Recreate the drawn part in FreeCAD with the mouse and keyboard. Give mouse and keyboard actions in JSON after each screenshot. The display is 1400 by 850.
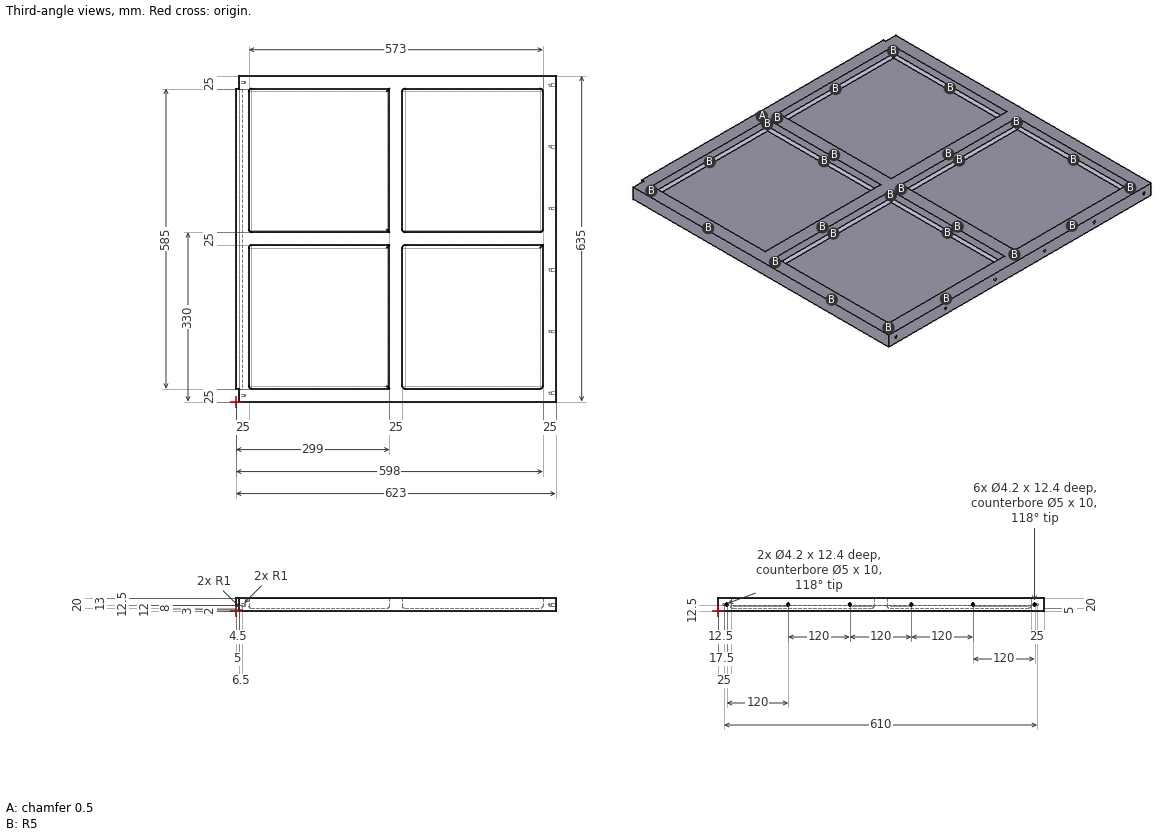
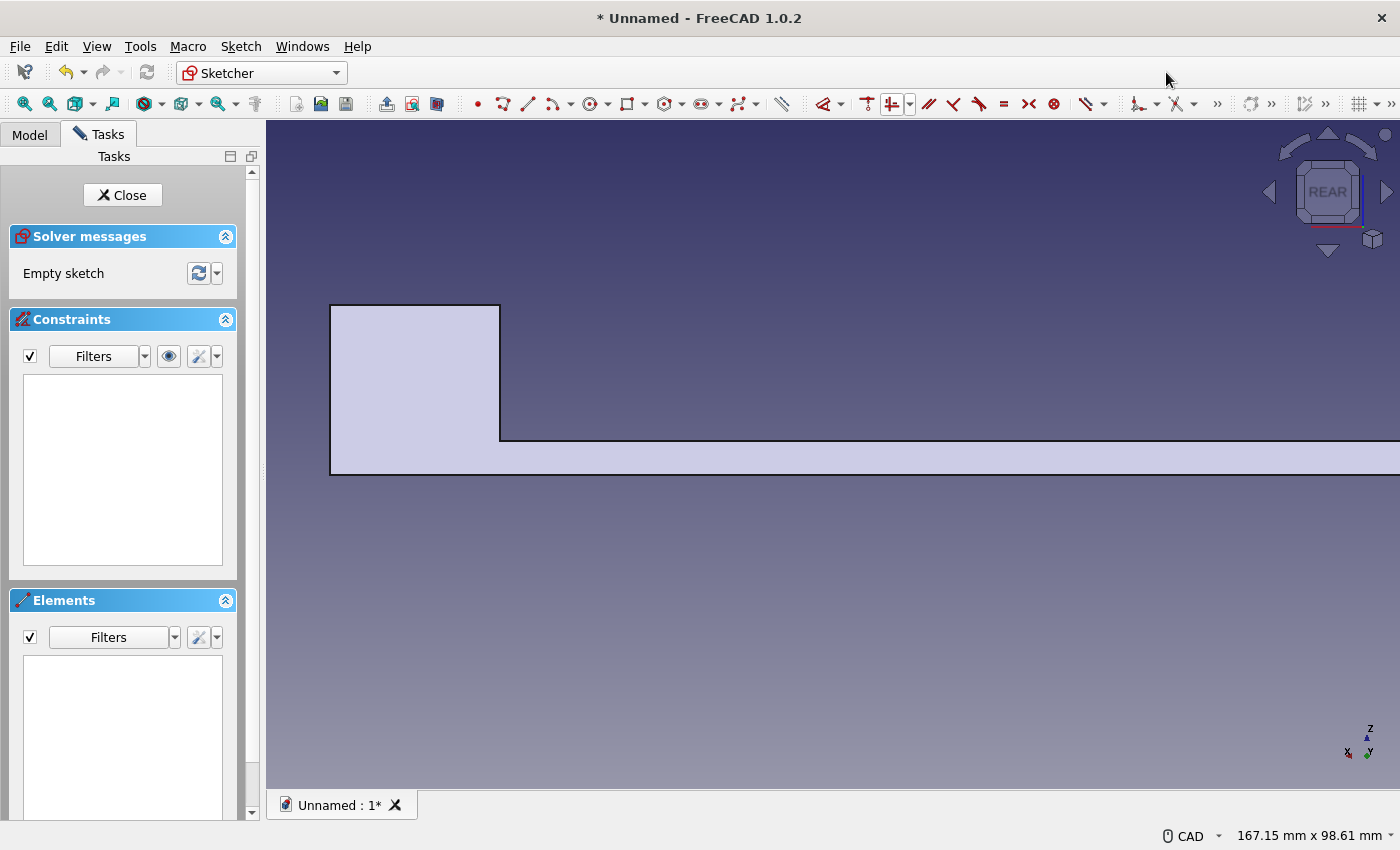
{"action": "scroll", "coordinate": [764, 454], "scroll_direction": "down", "scroll_amount": 5}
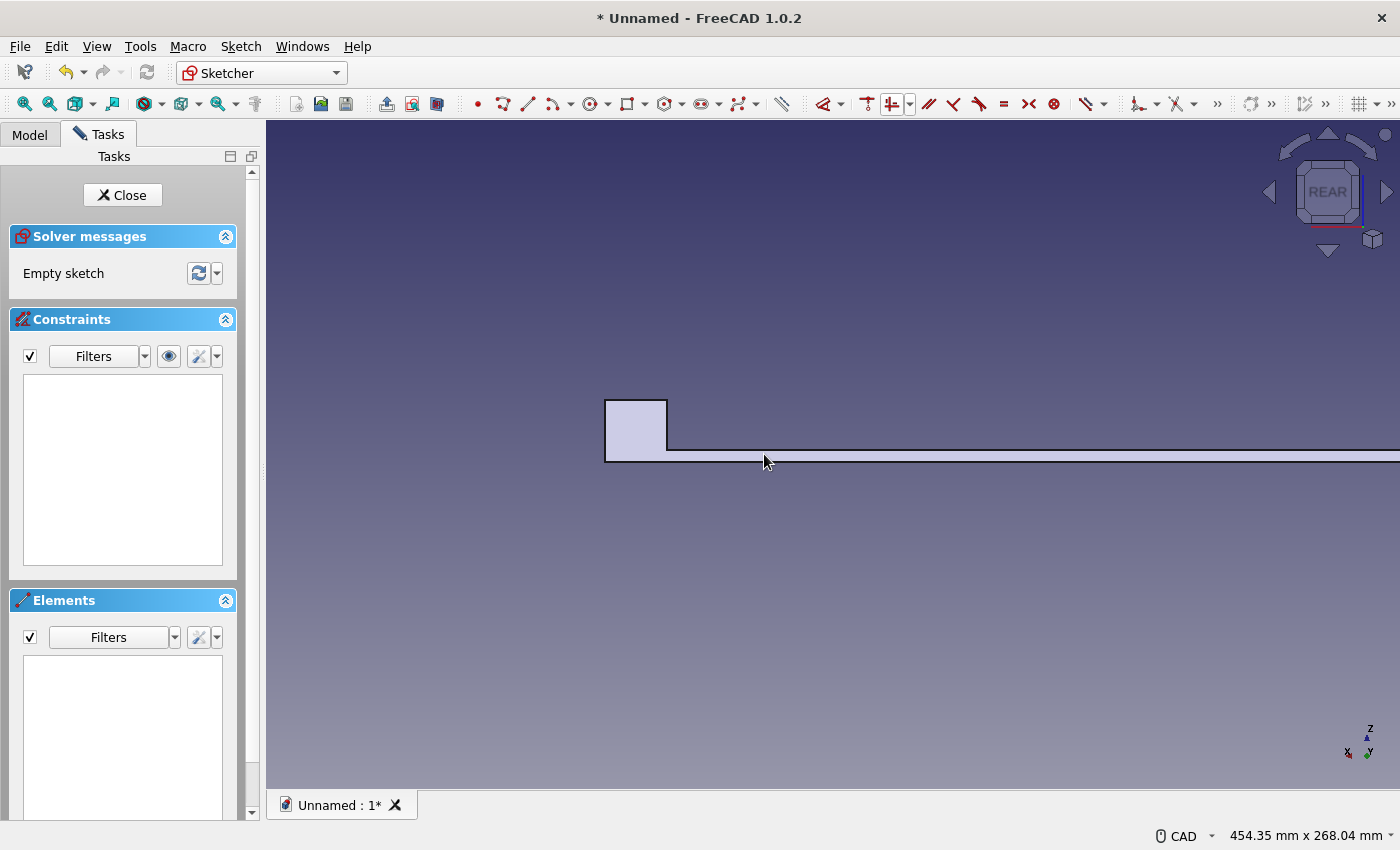
{"action": "scroll", "coordinate": [764, 454], "scroll_direction": "down", "scroll_amount": 5}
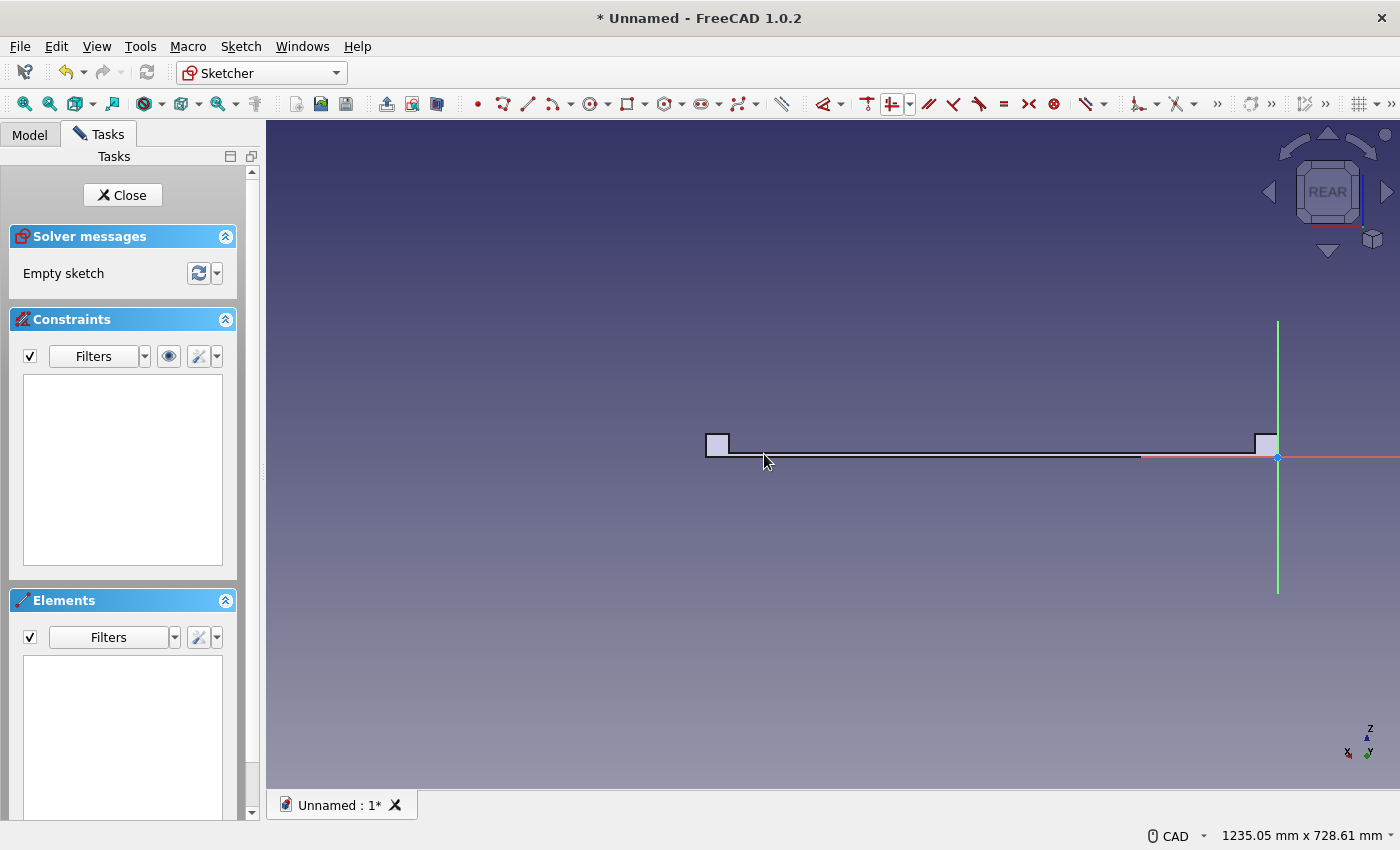
{"action": "scroll", "coordinate": [764, 454], "scroll_direction": "down", "scroll_amount": 5}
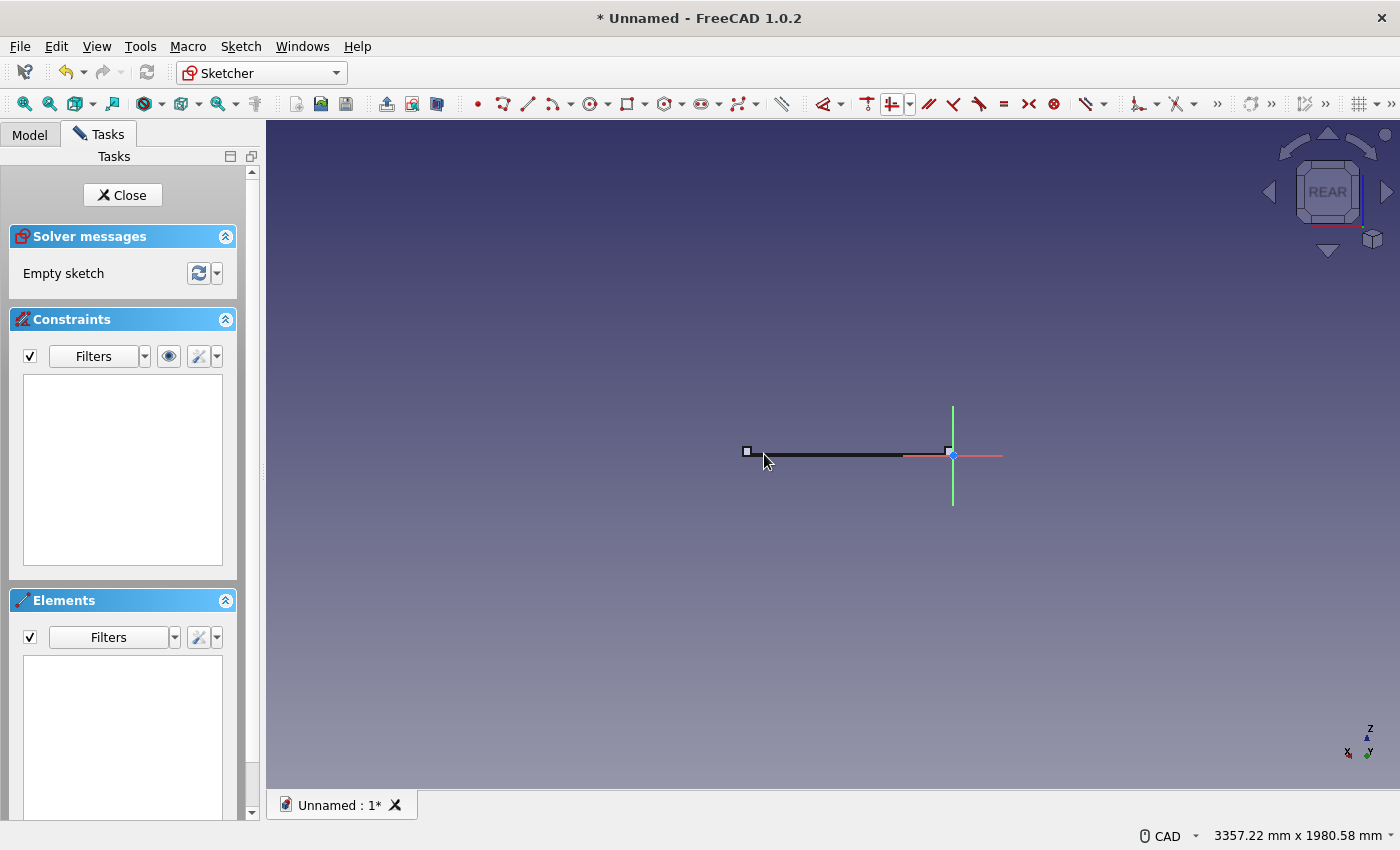
{"action": "scroll", "coordinate": [961, 453], "scroll_direction": "up", "scroll_amount": 15}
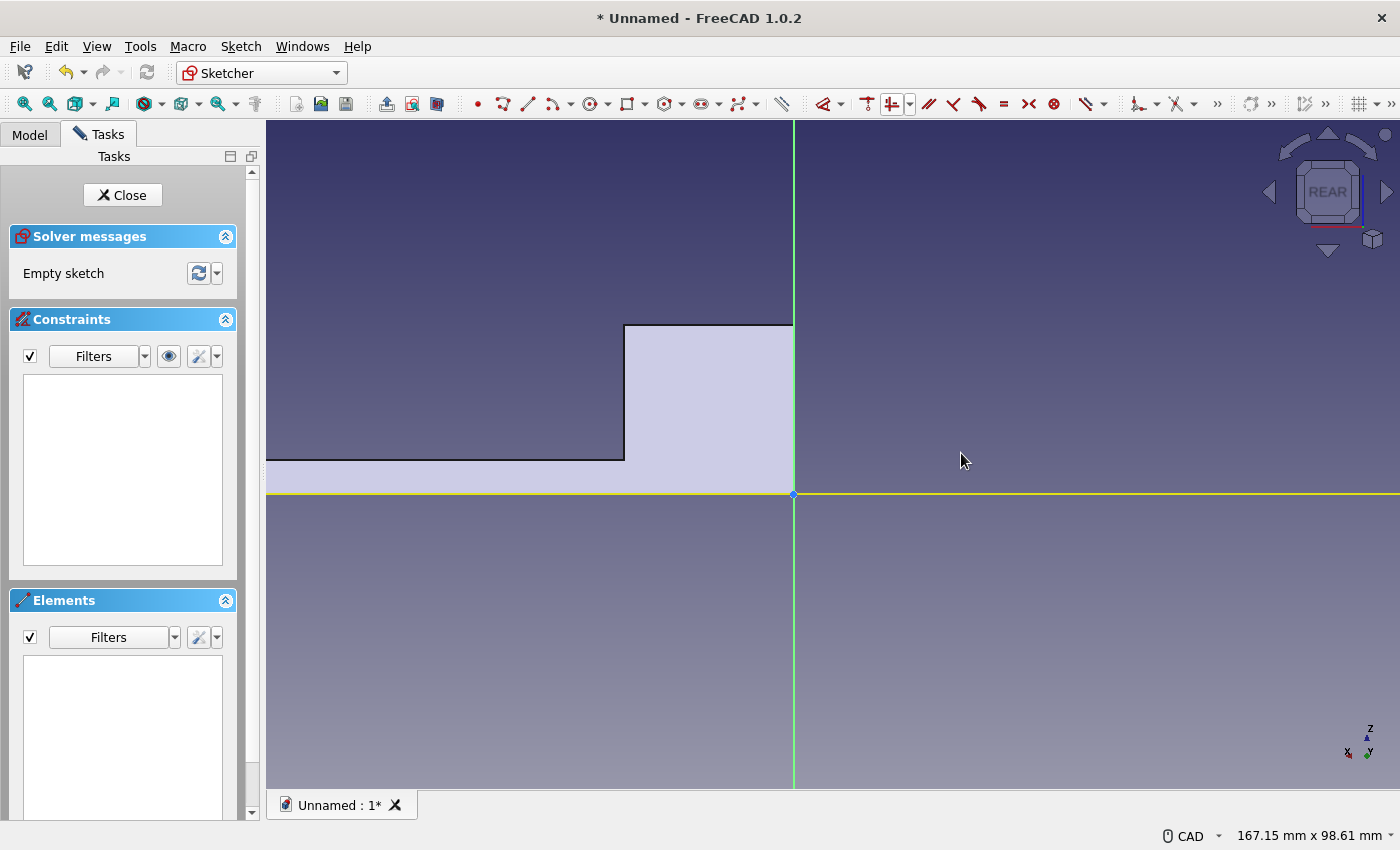
{"action": "scroll", "coordinate": [748, 453], "scroll_direction": "up", "scroll_amount": 8}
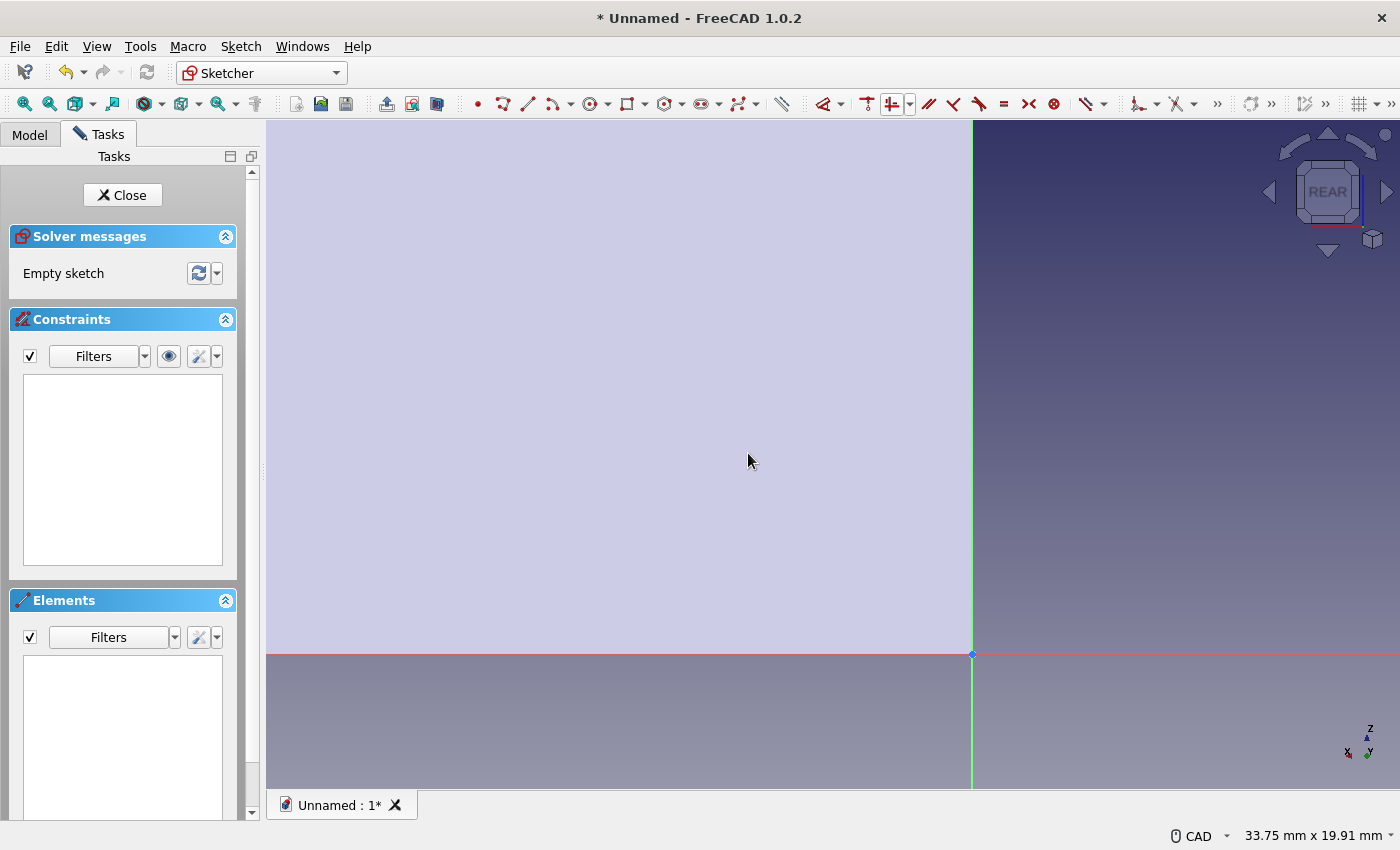
{"action": "key", "text": "g l"}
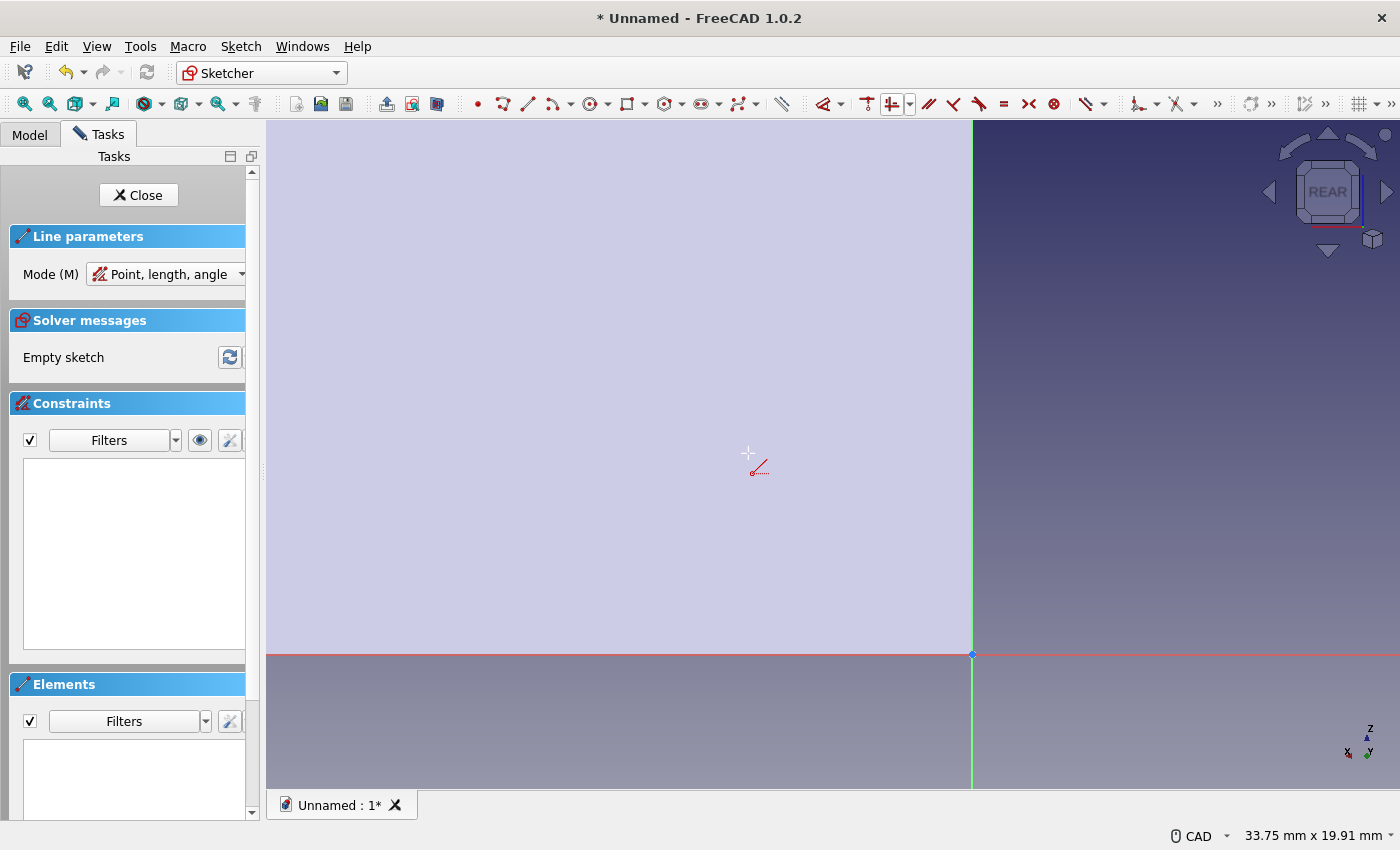
{"action": "left_click", "coordinate": [552, 285]}
{"action": "left_click", "coordinate": [552, 554]}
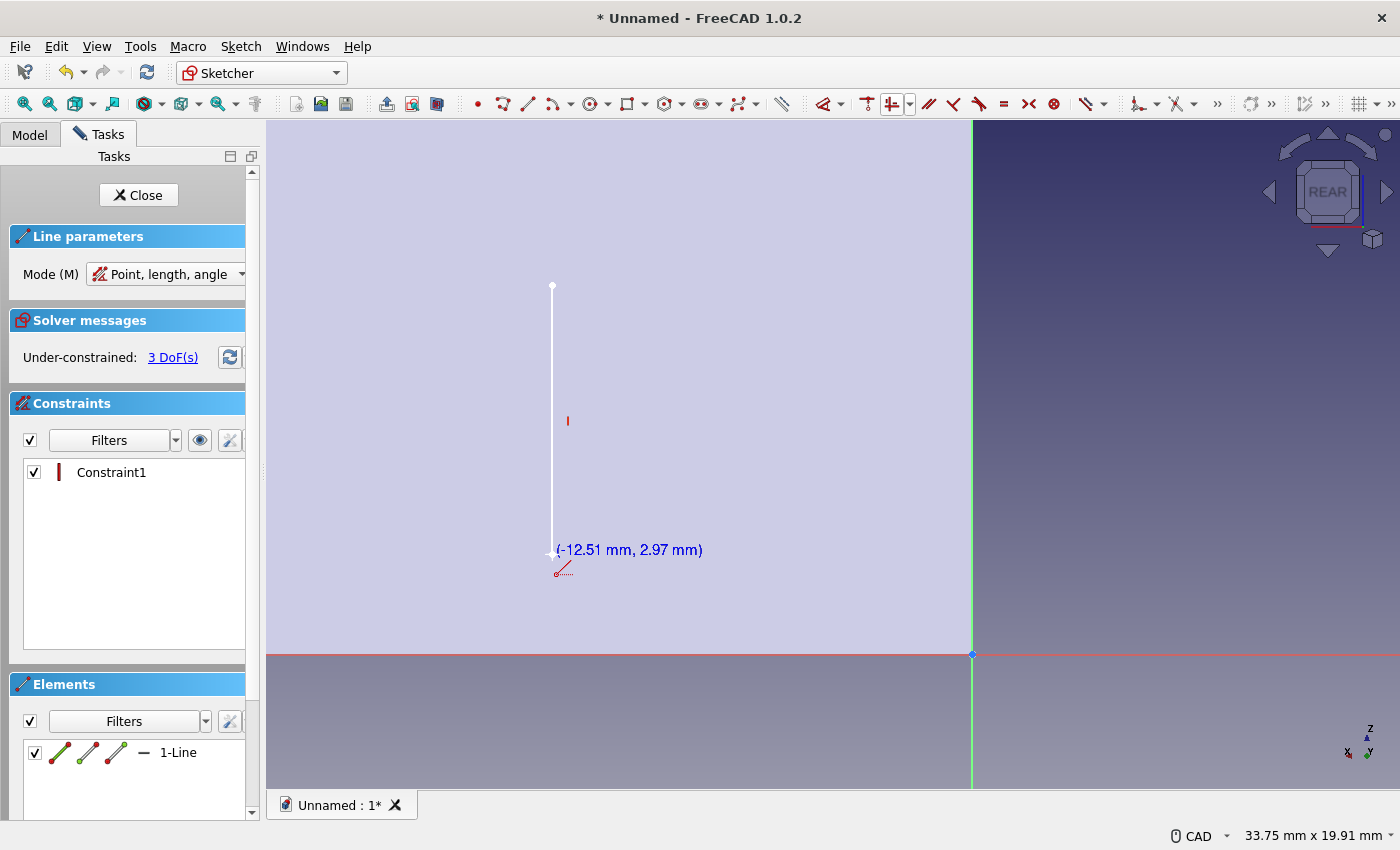
{"action": "key", "text": "g m"}